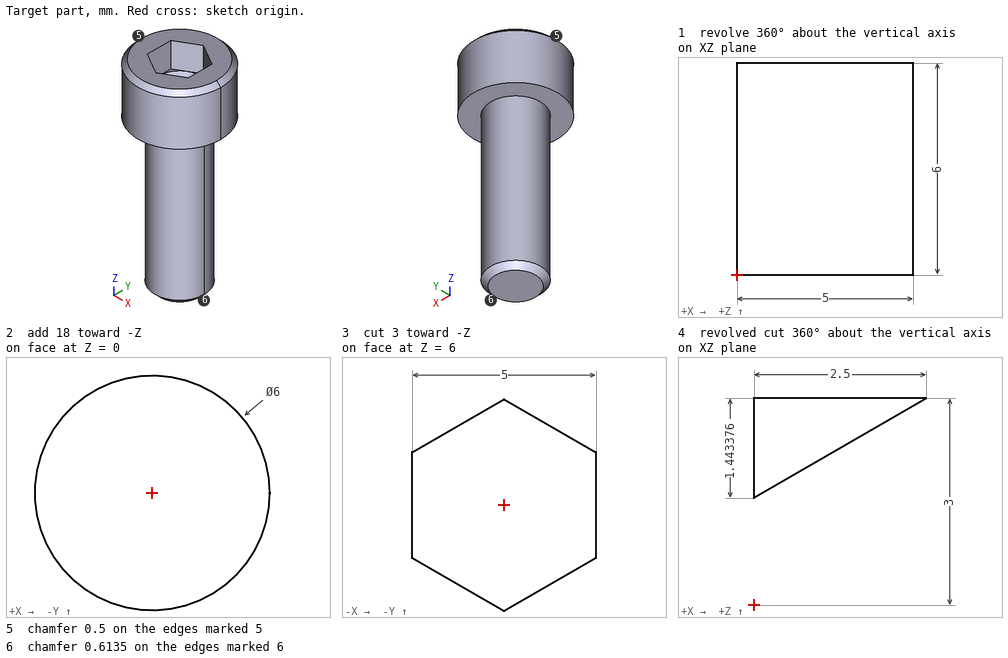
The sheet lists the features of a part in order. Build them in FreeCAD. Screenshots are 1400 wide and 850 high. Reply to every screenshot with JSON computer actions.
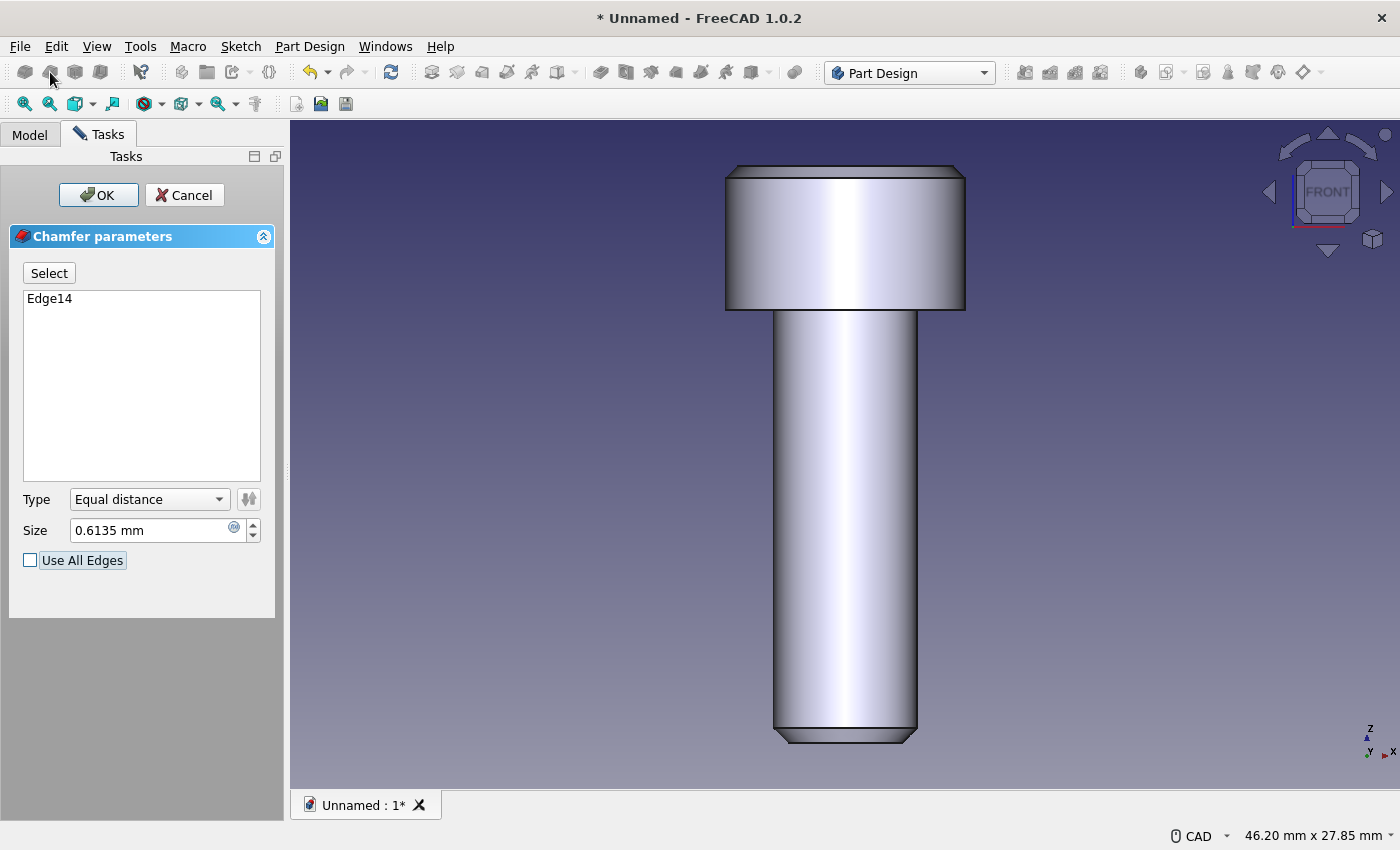
{"action": "left_click", "coordinate": [99, 195]}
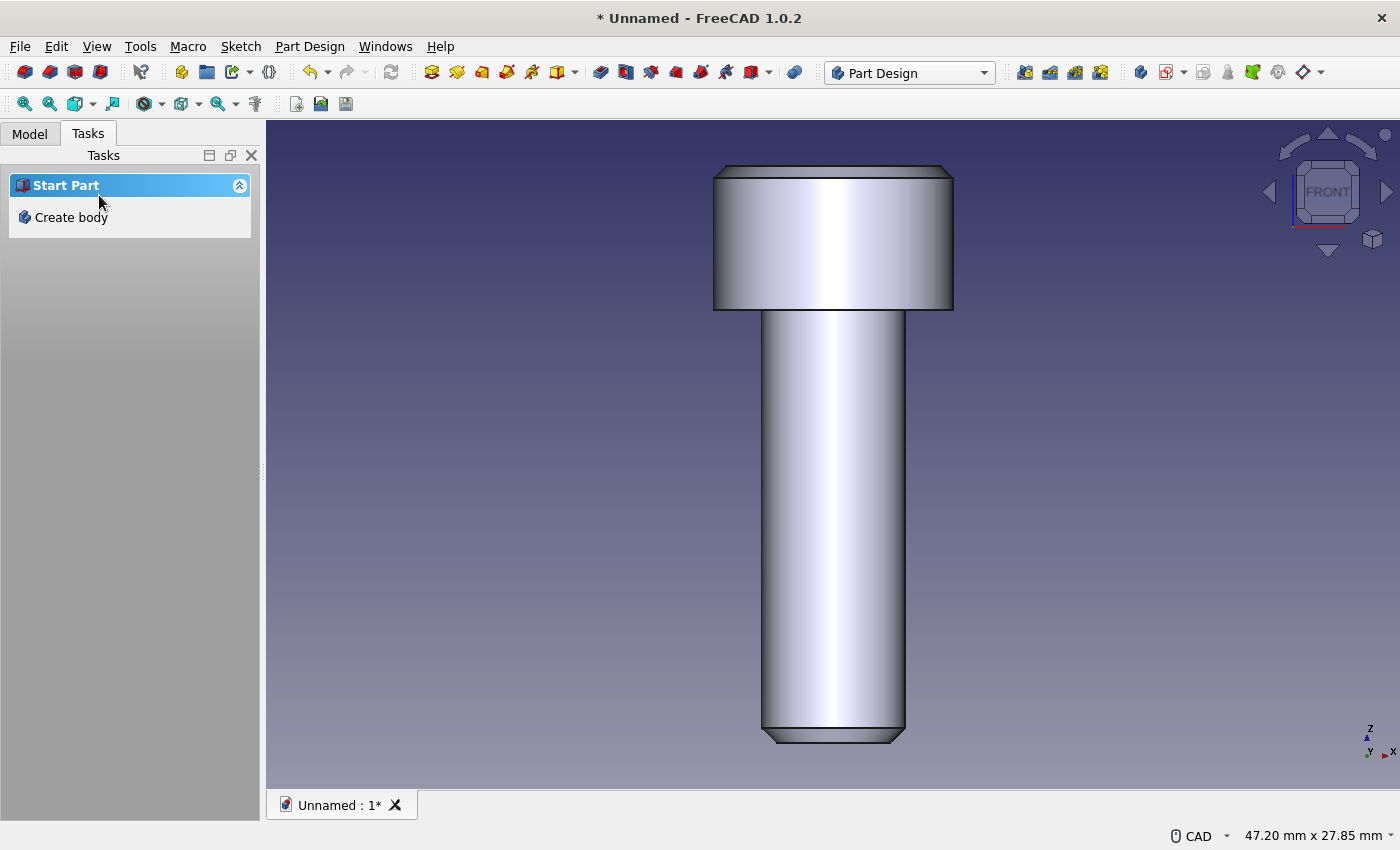
{"action": "key", "text": "0"}